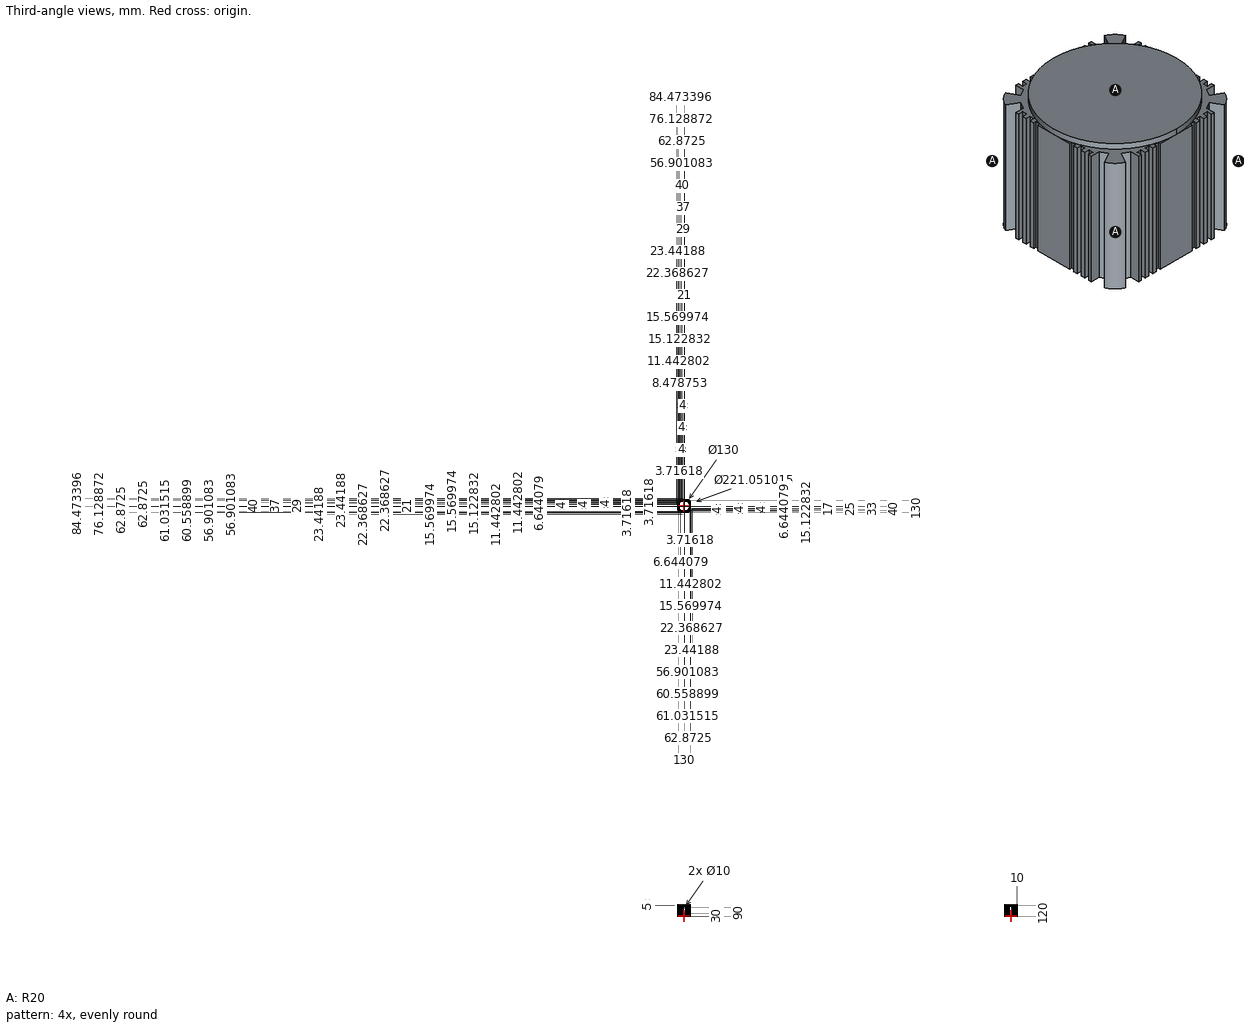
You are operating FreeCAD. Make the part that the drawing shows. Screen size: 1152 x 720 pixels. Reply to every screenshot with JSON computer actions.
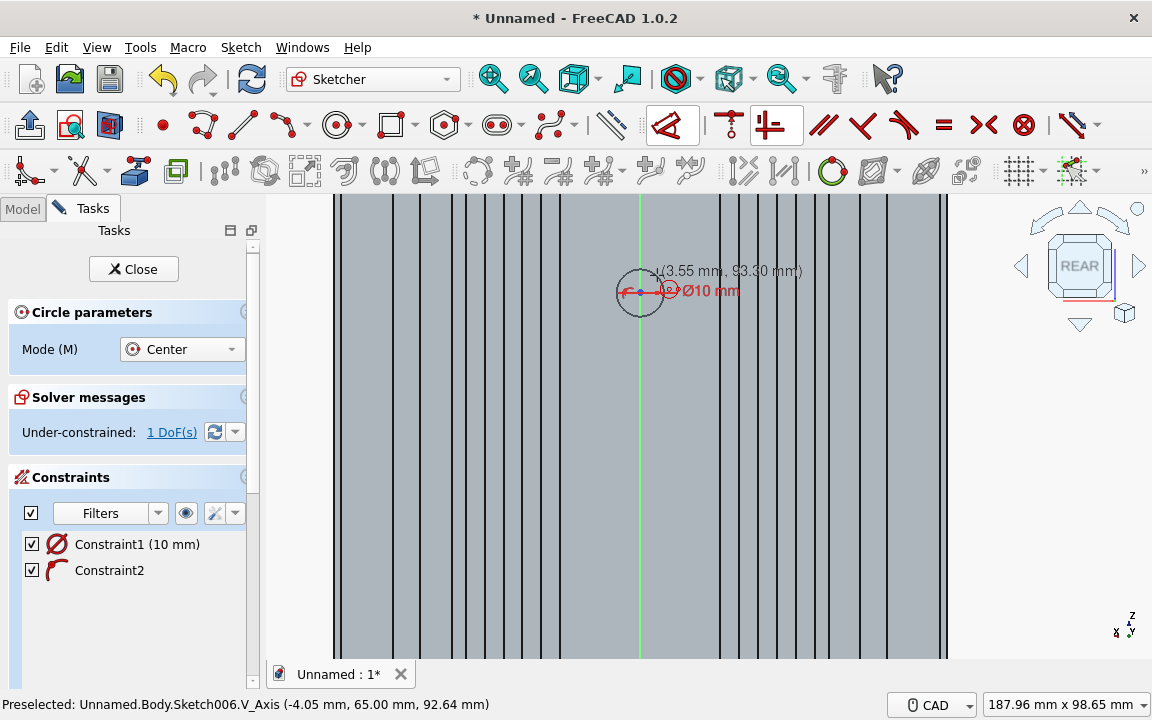
{"action": "left_click", "coordinate": [640, 574]}
{"action": "mouse_move", "coordinate": [657, 558]}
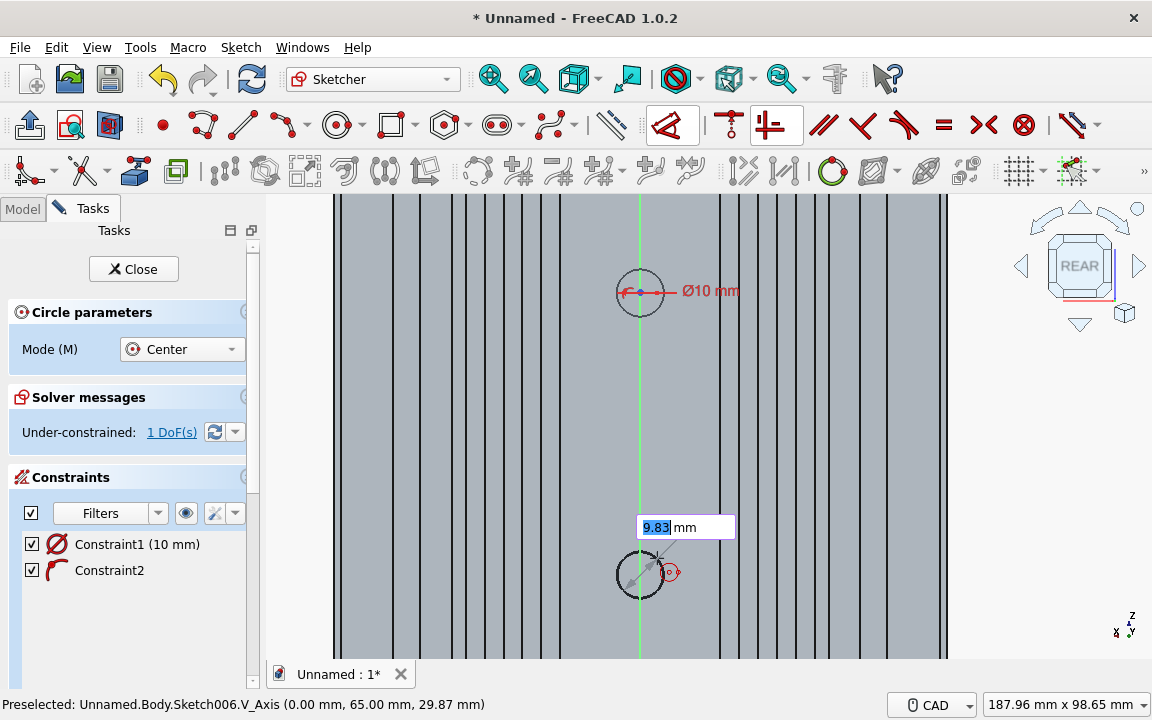
{"action": "type", "text": "10"}
{"action": "key", "text": "Return"}
{"action": "key", "text": "Escape"}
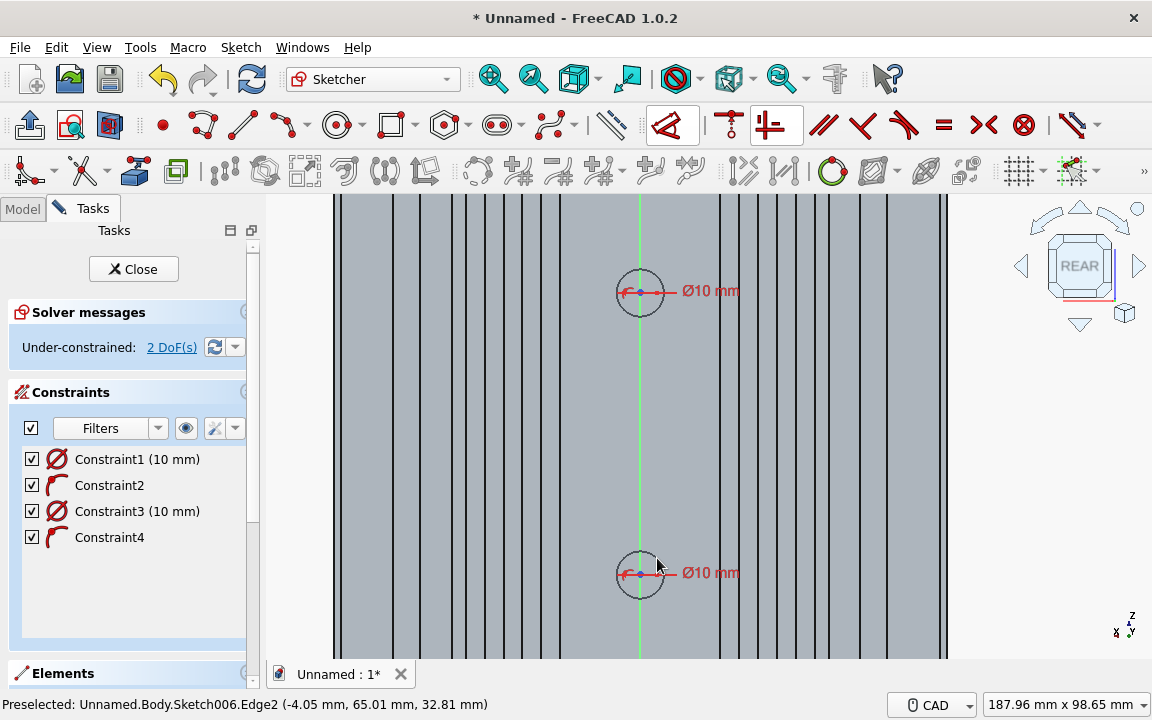
{"action": "left_click", "coordinate": [640, 293]}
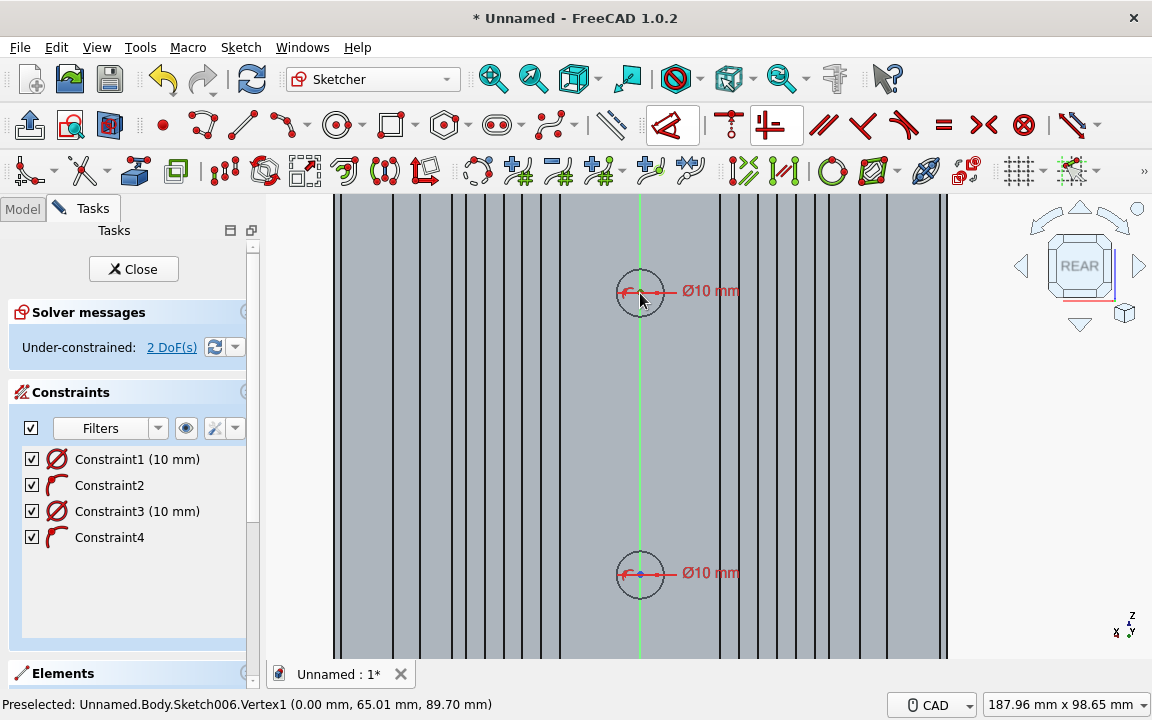
{"action": "key", "text": "i"}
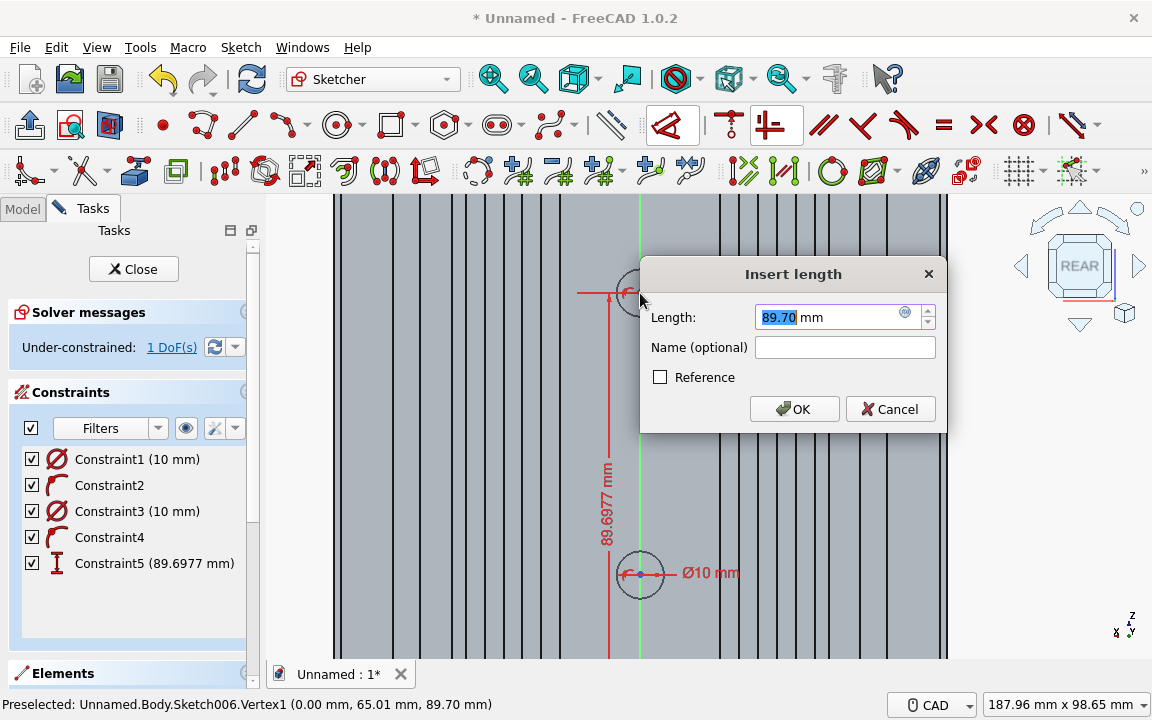
{"action": "type", "text": "90"}
{"action": "key", "text": "Return"}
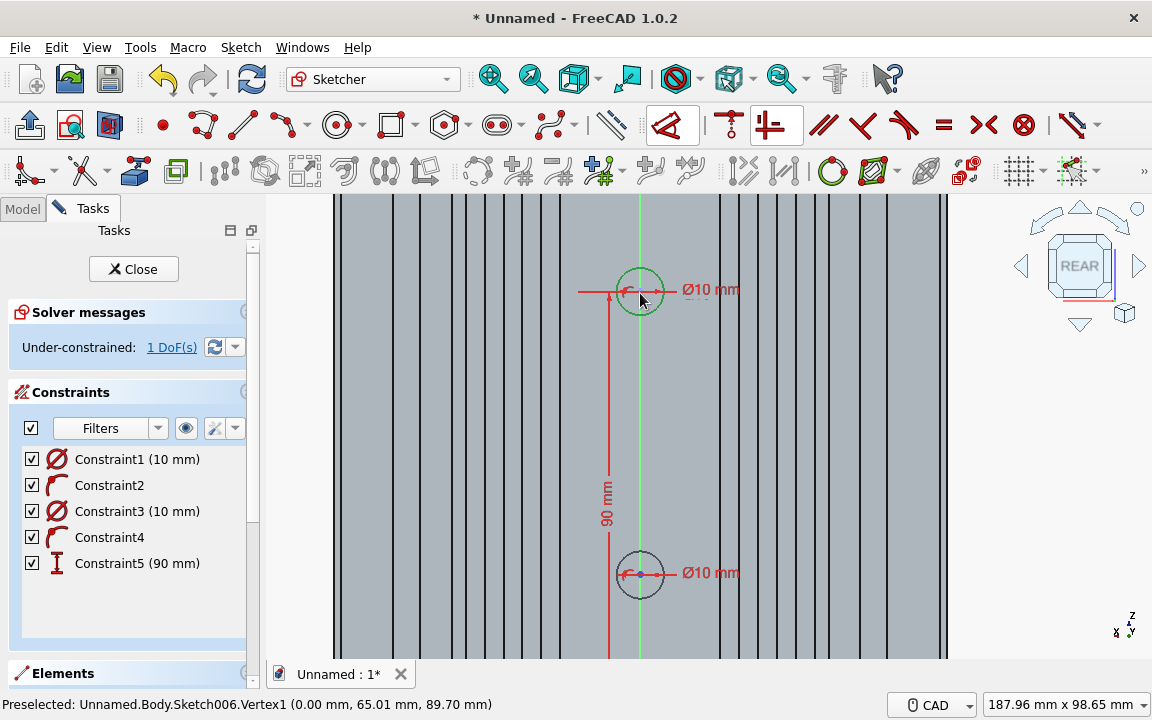
{"action": "left_click", "coordinate": [640, 575]}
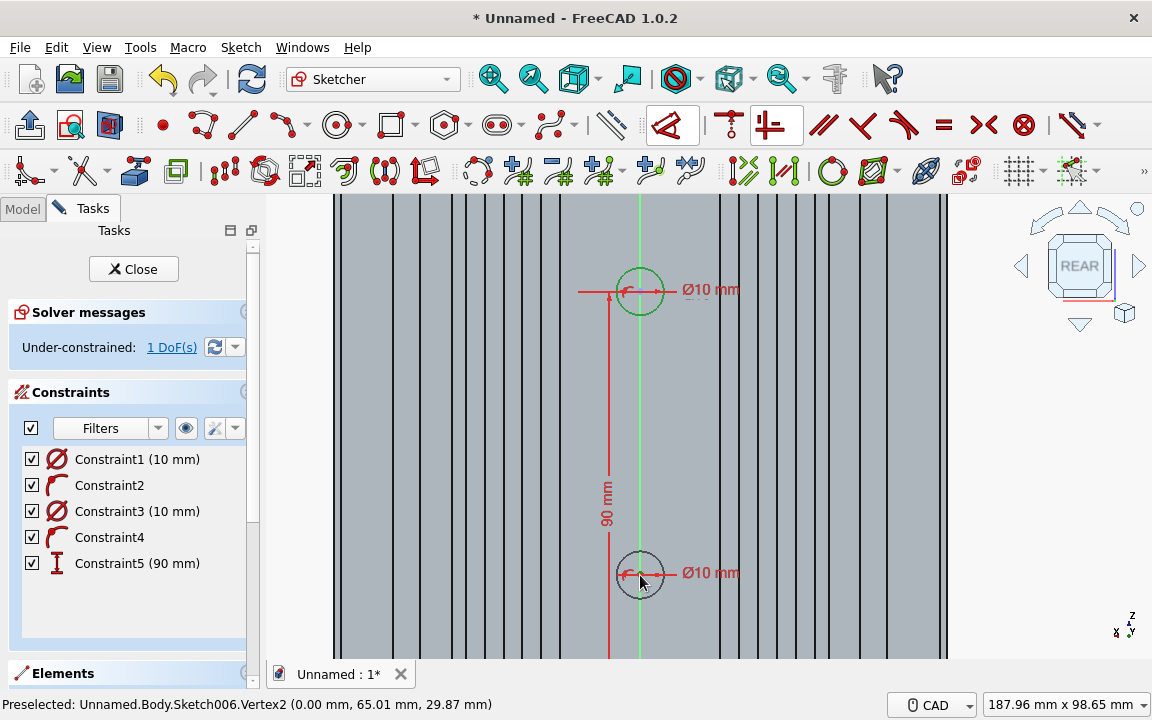
{"action": "left_click", "coordinate": [694, 126]}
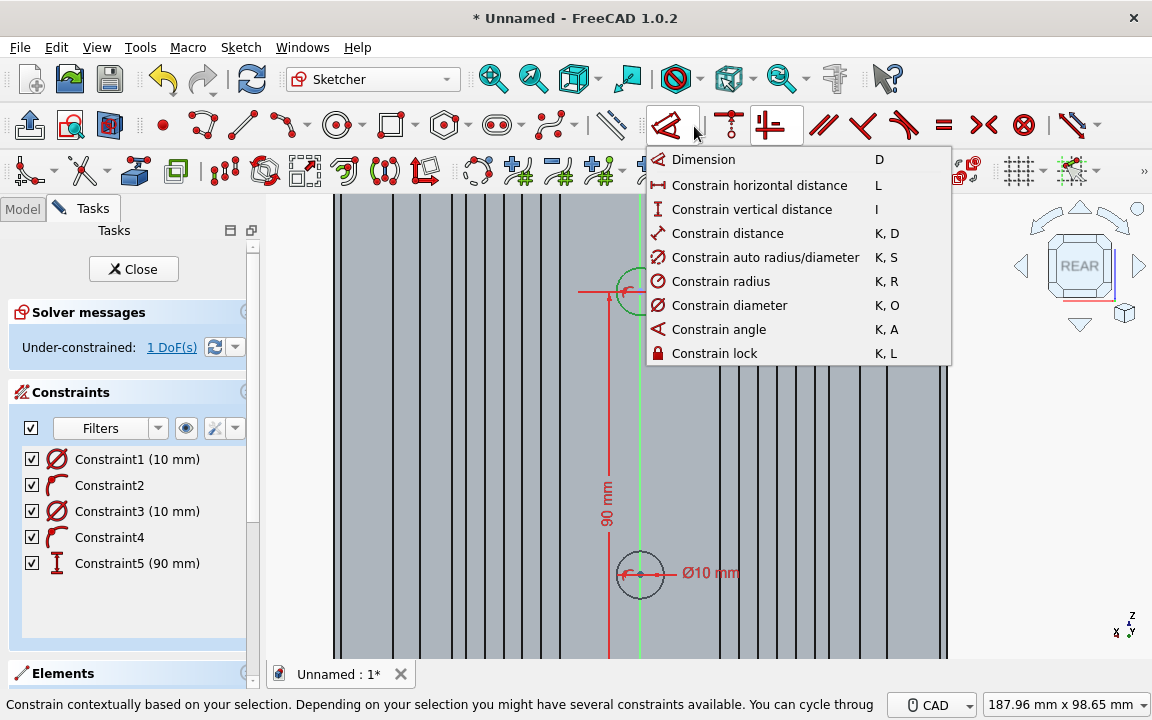
{"action": "left_click", "coordinate": [799, 209]}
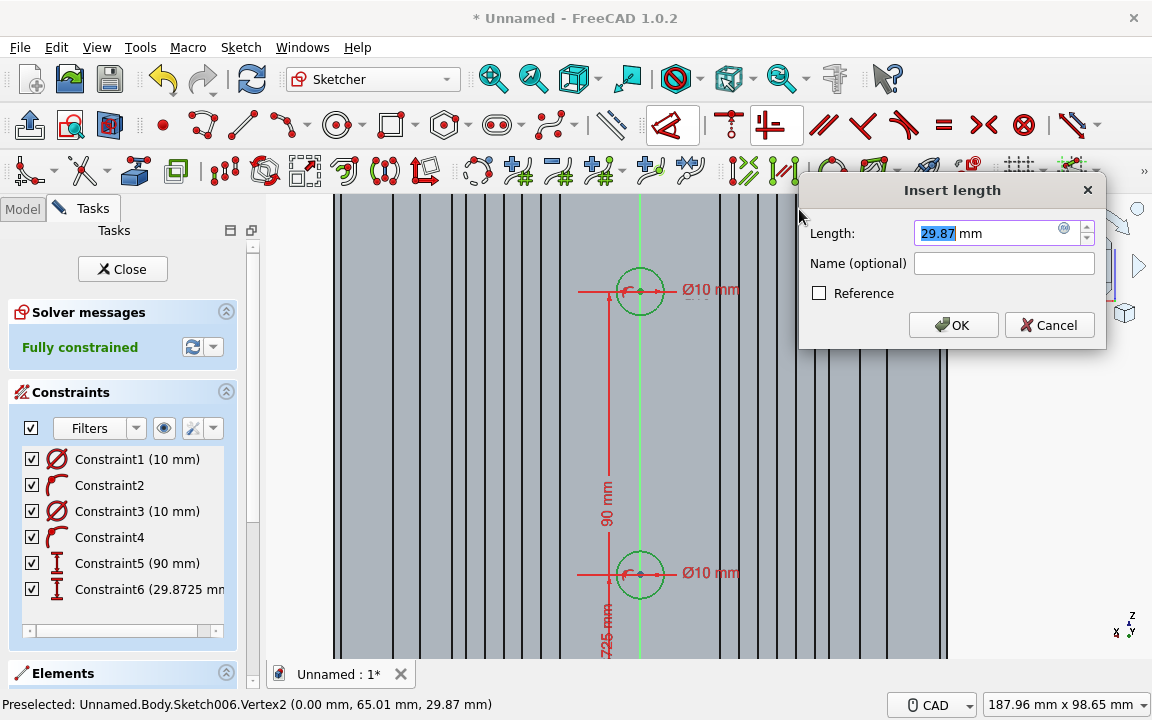
{"action": "type", "text": "30"}
{"action": "key", "text": "Return"}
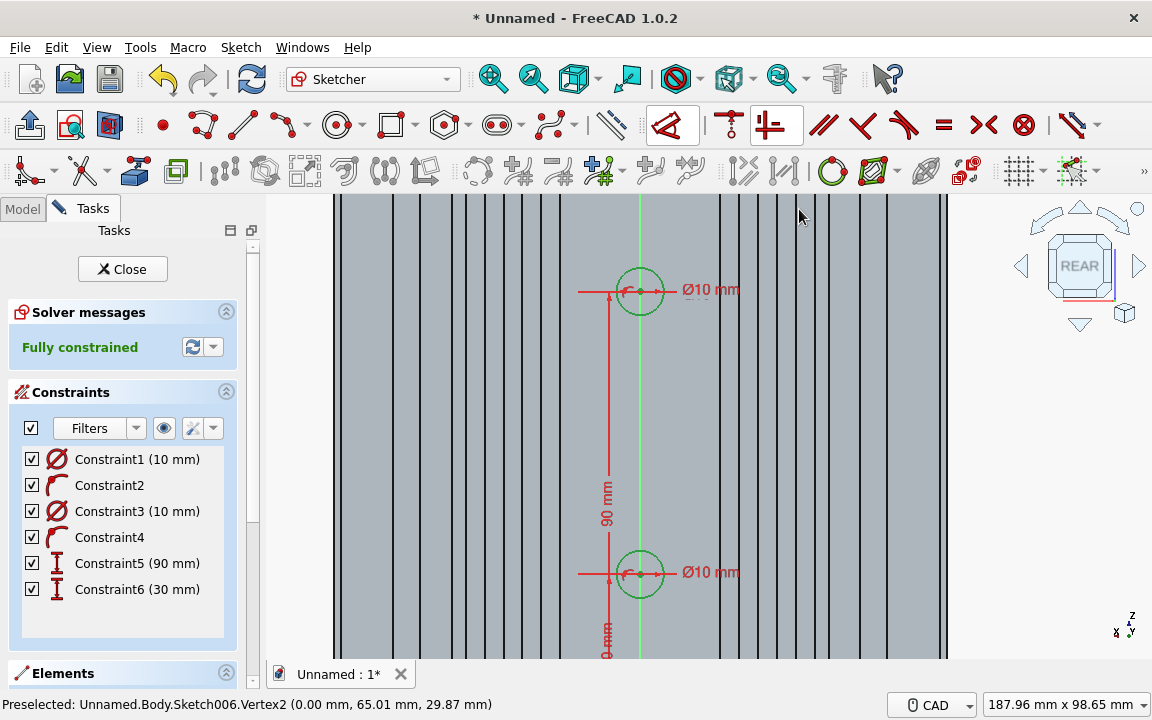
{"action": "left_click", "coordinate": [123, 269]}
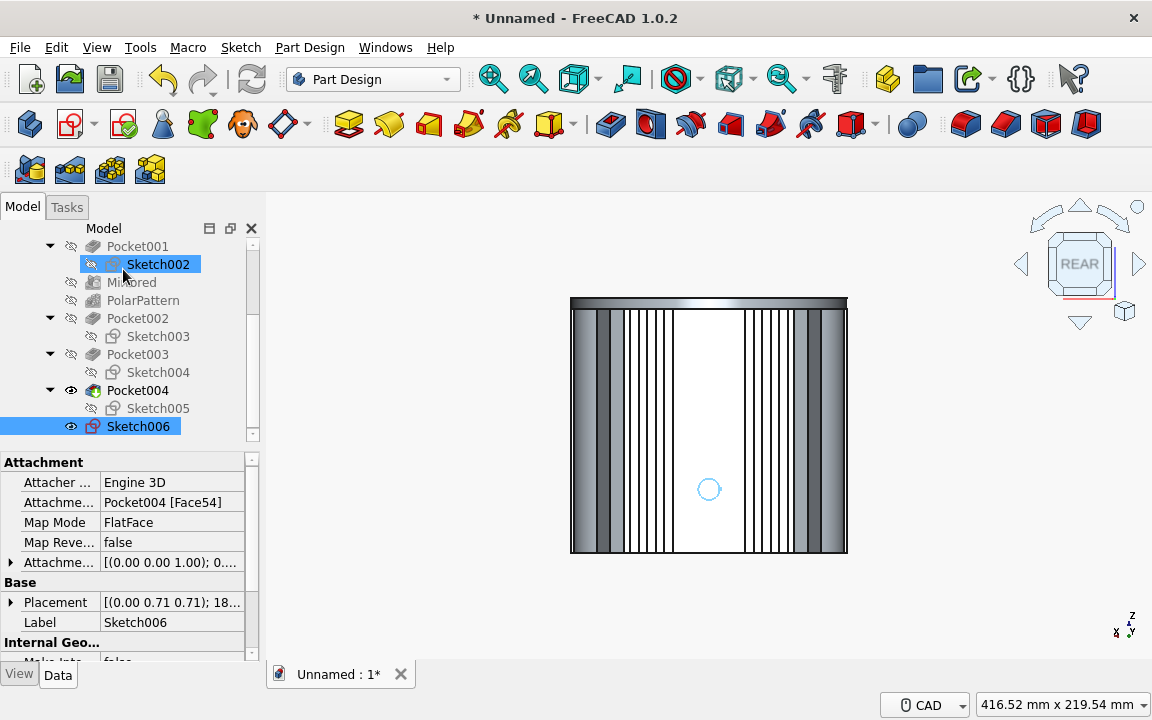
{"action": "left_click", "coordinate": [612, 124]}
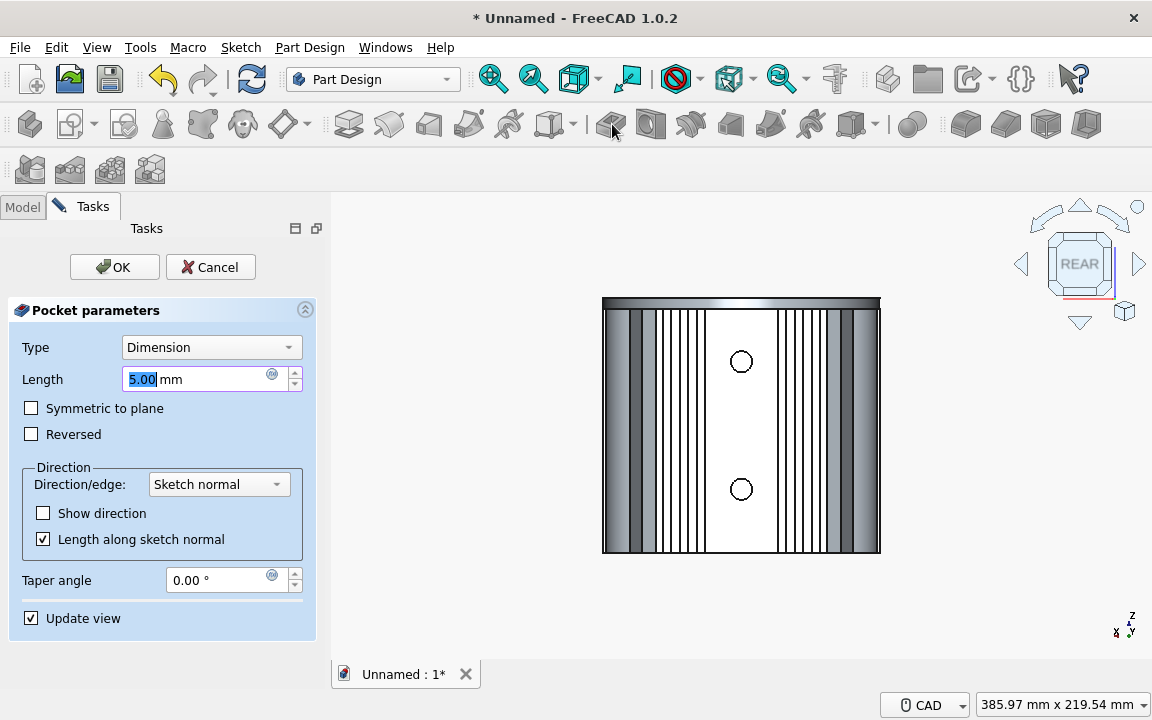
{"action": "type", "text": "10"}
{"action": "key", "text": "Tab"}